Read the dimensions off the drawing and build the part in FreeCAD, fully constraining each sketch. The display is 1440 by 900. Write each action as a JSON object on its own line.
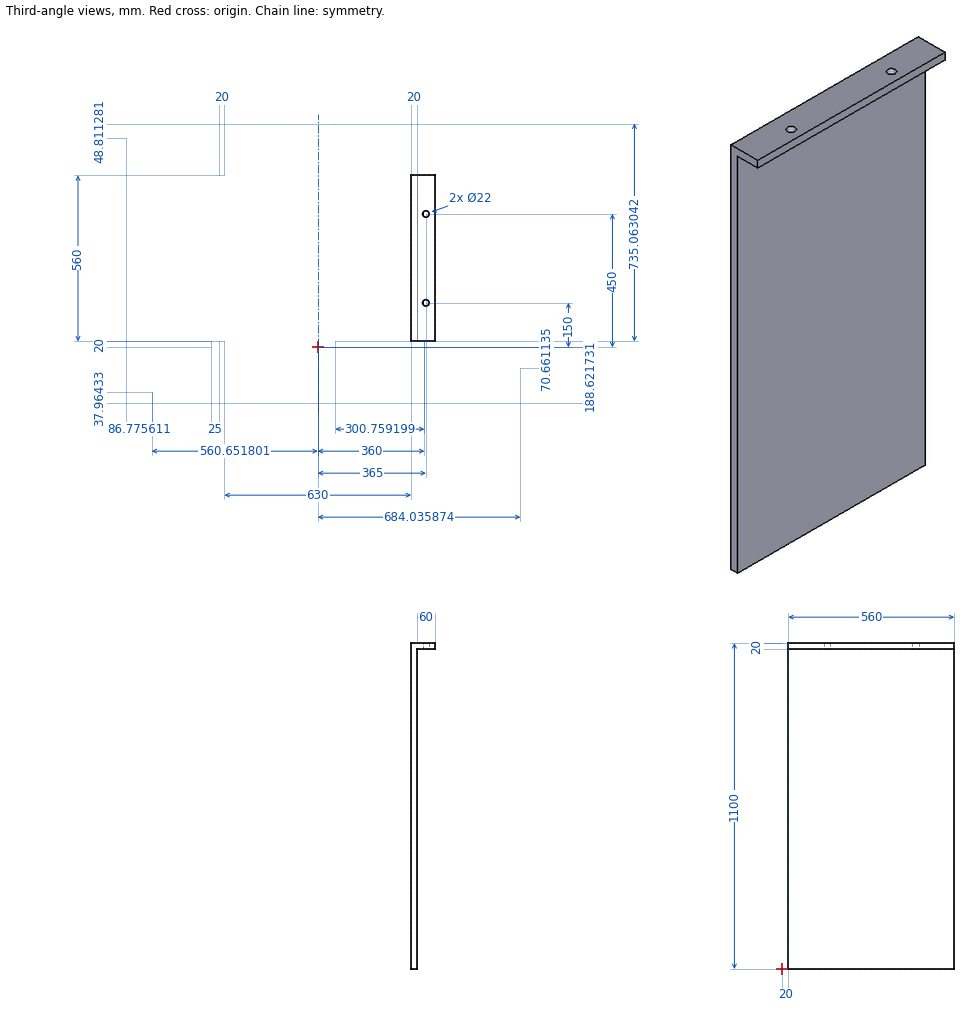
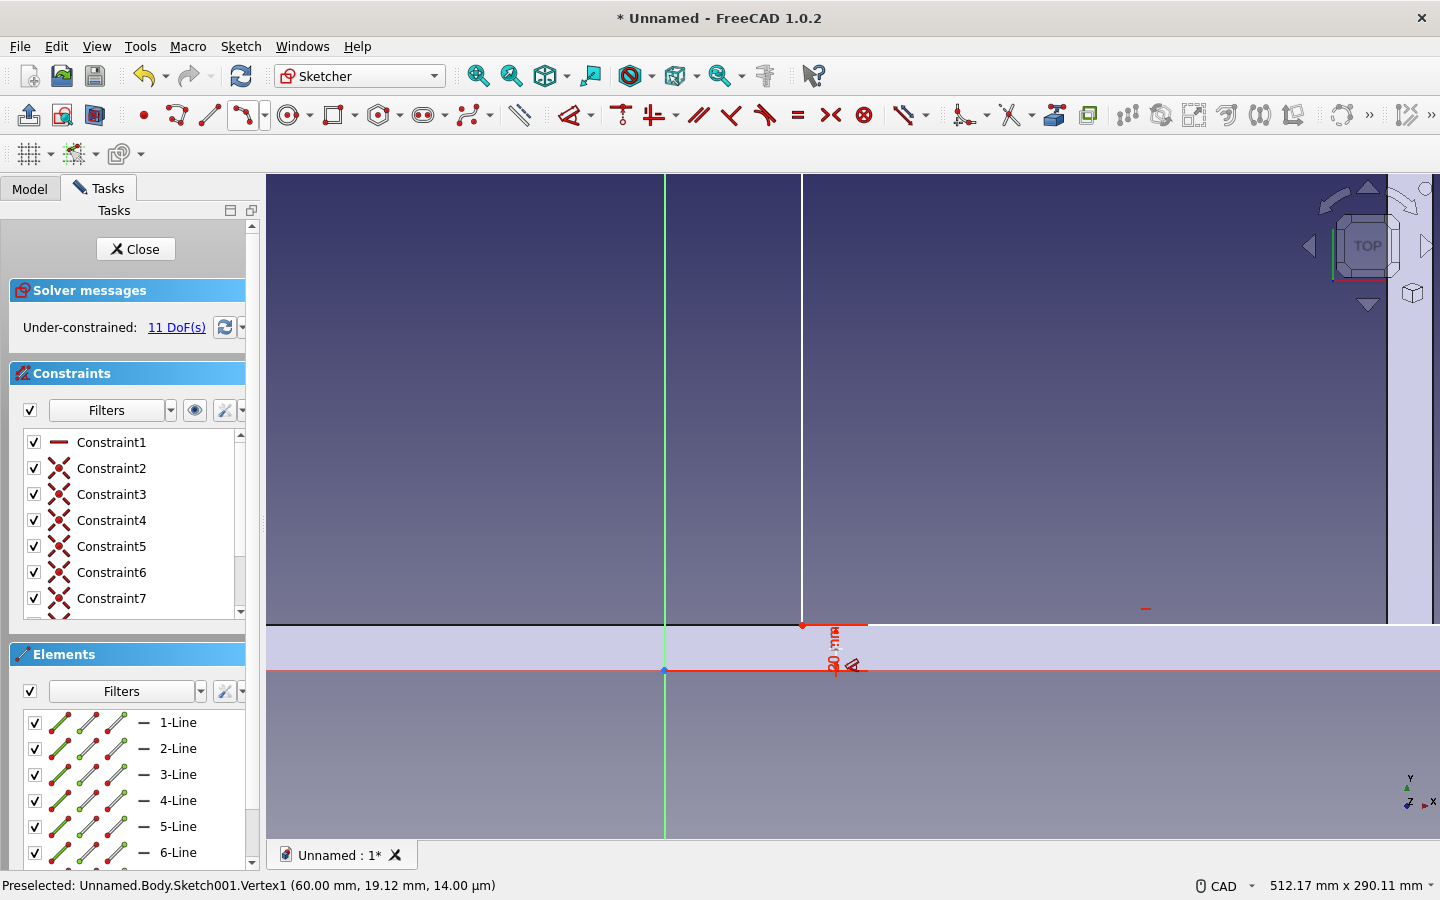
{"action": "scroll", "coordinate": [804, 629], "scroll_direction": "down", "scroll_amount": 8}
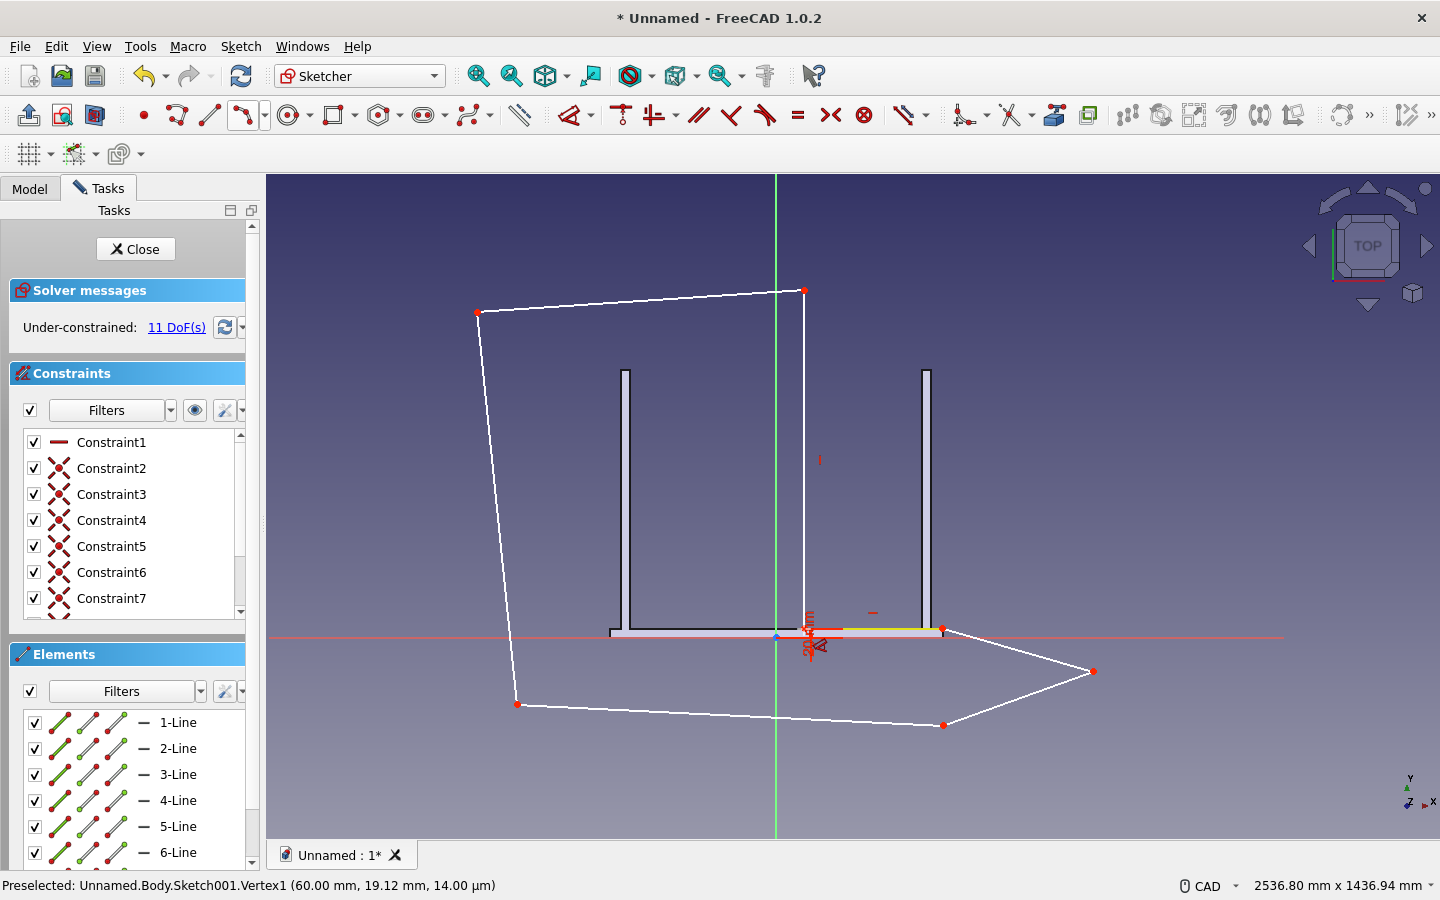
{"action": "left_click", "coordinate": [943, 629]}
{"action": "left_click", "coordinate": [860, 672]}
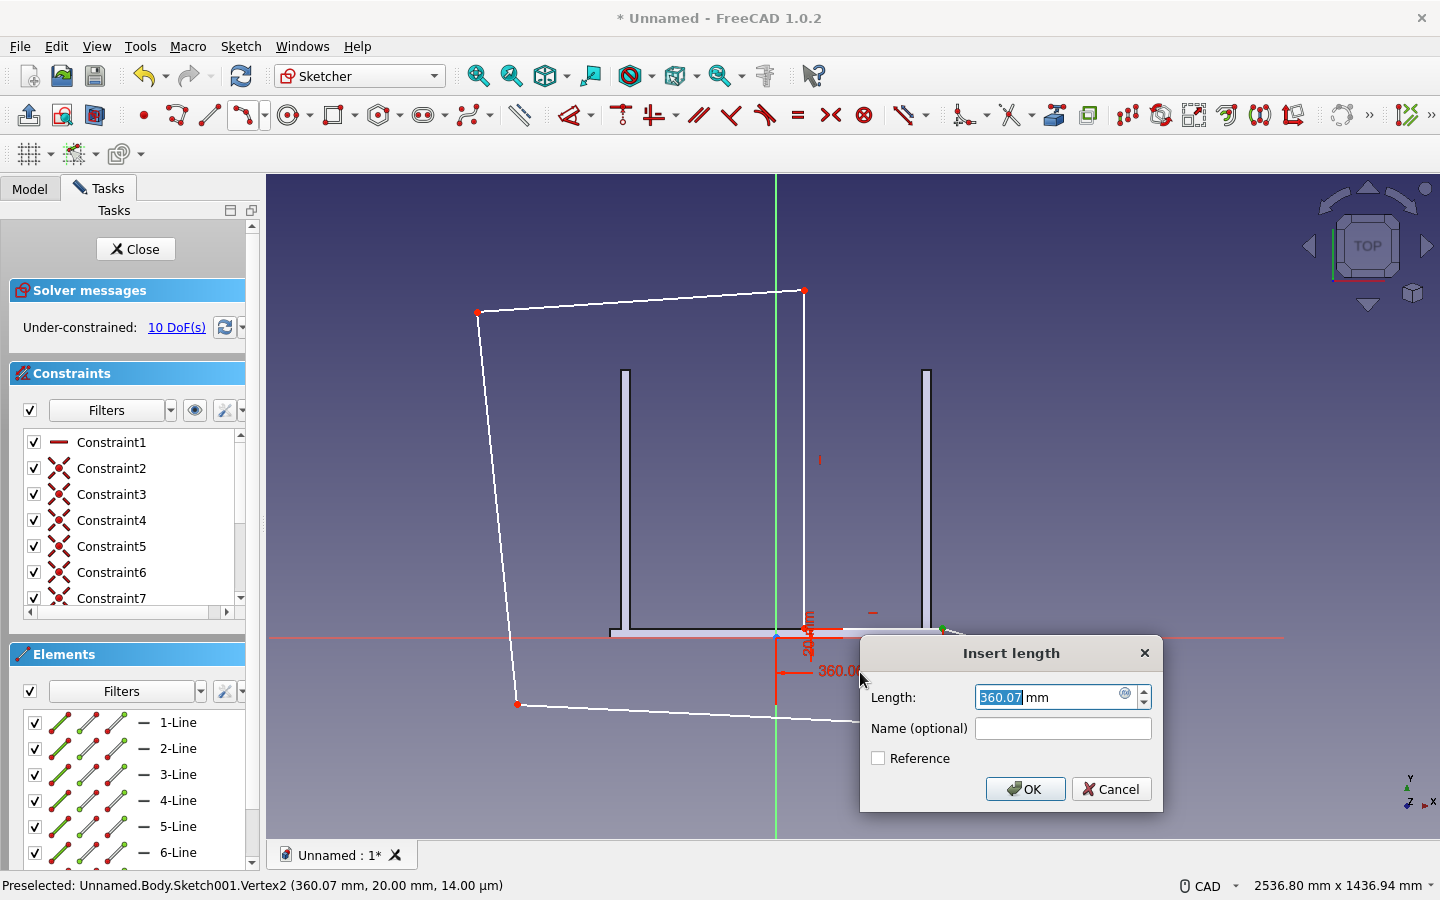
{"action": "type", "text": "360"}
{"action": "key", "text": "Return"}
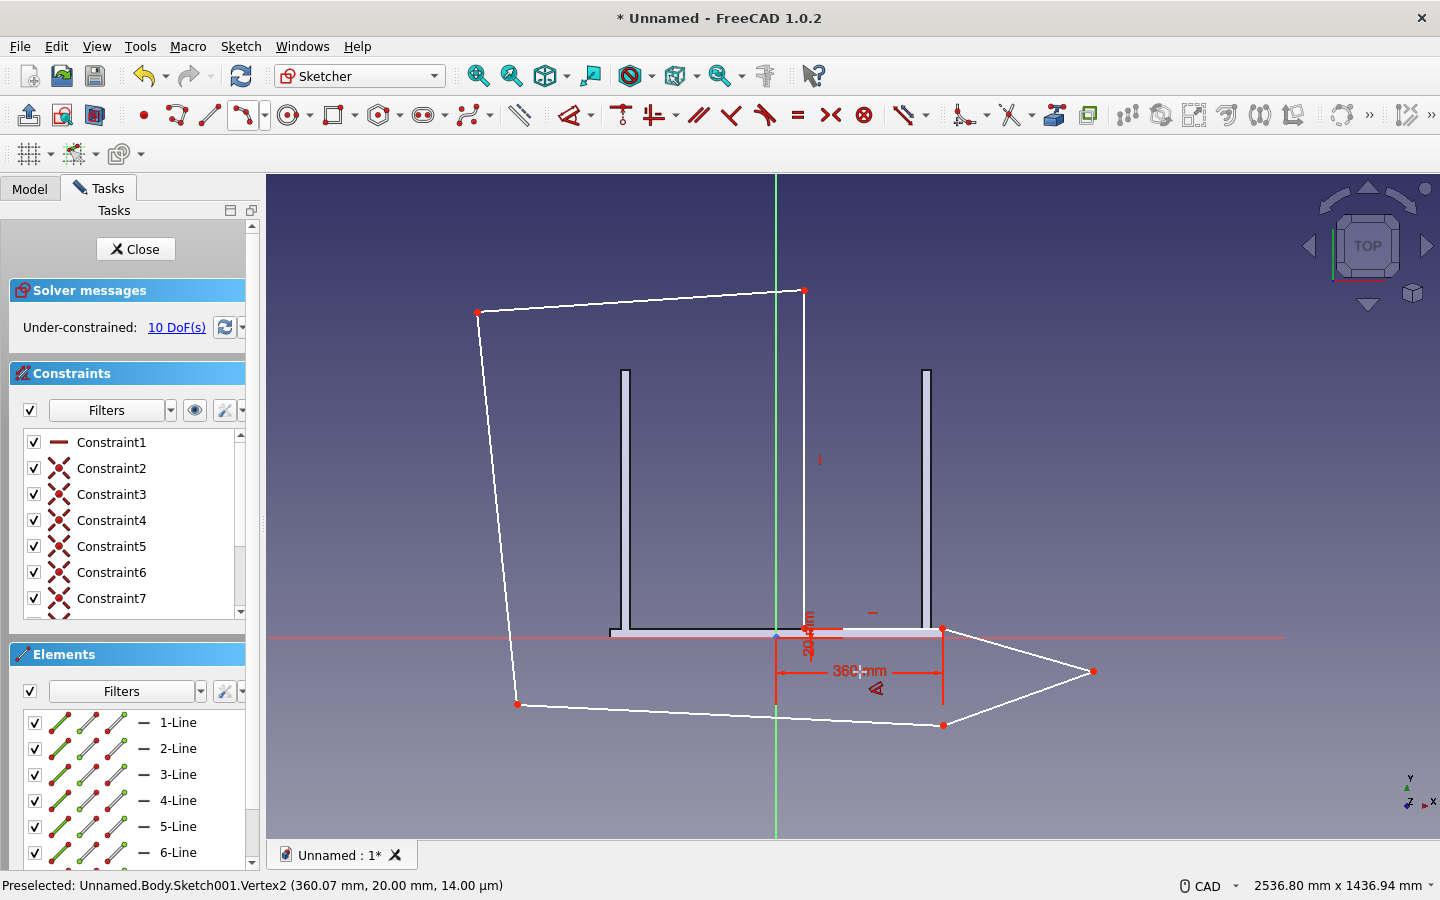
{"action": "left_click", "coordinate": [943, 726]}
{"action": "left_click", "coordinate": [860, 760]}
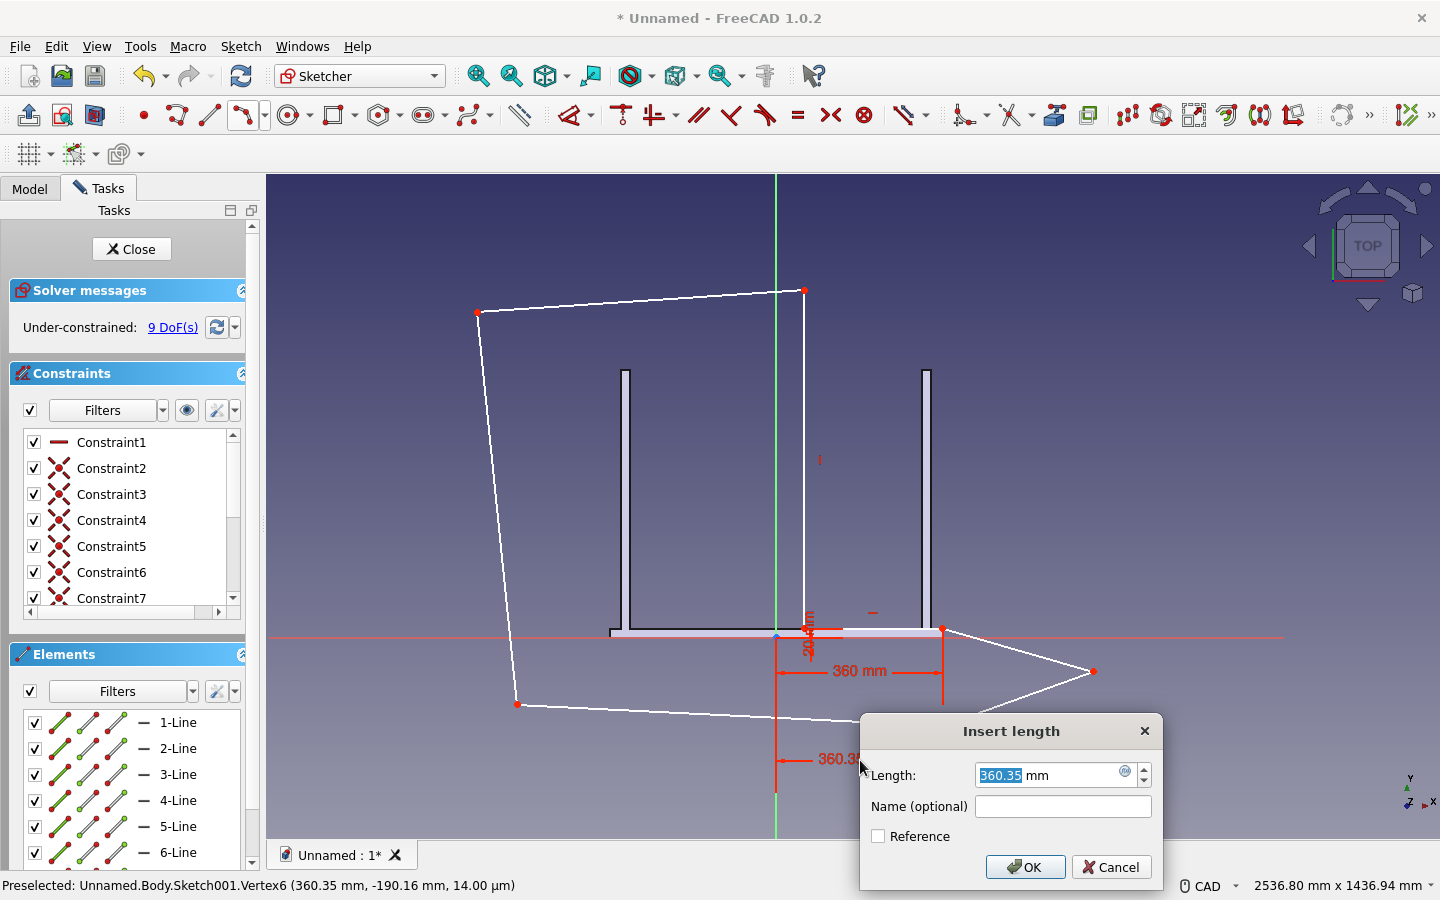
{"action": "type", "text": "360"}
{"action": "key", "text": "Return"}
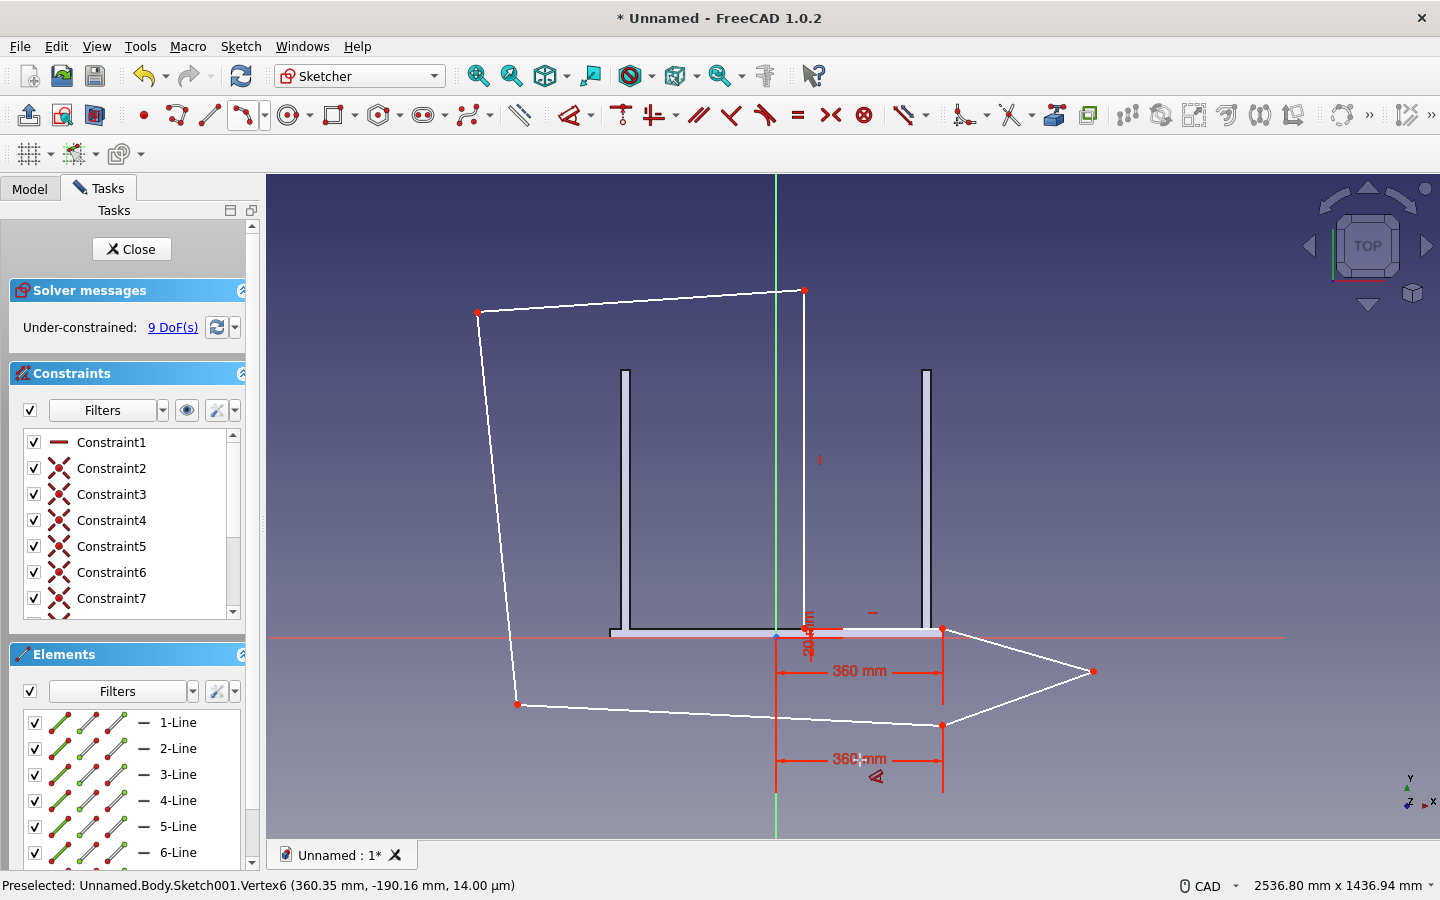
{"action": "scroll", "coordinate": [815, 720], "scroll_direction": "up", "scroll_amount": 5}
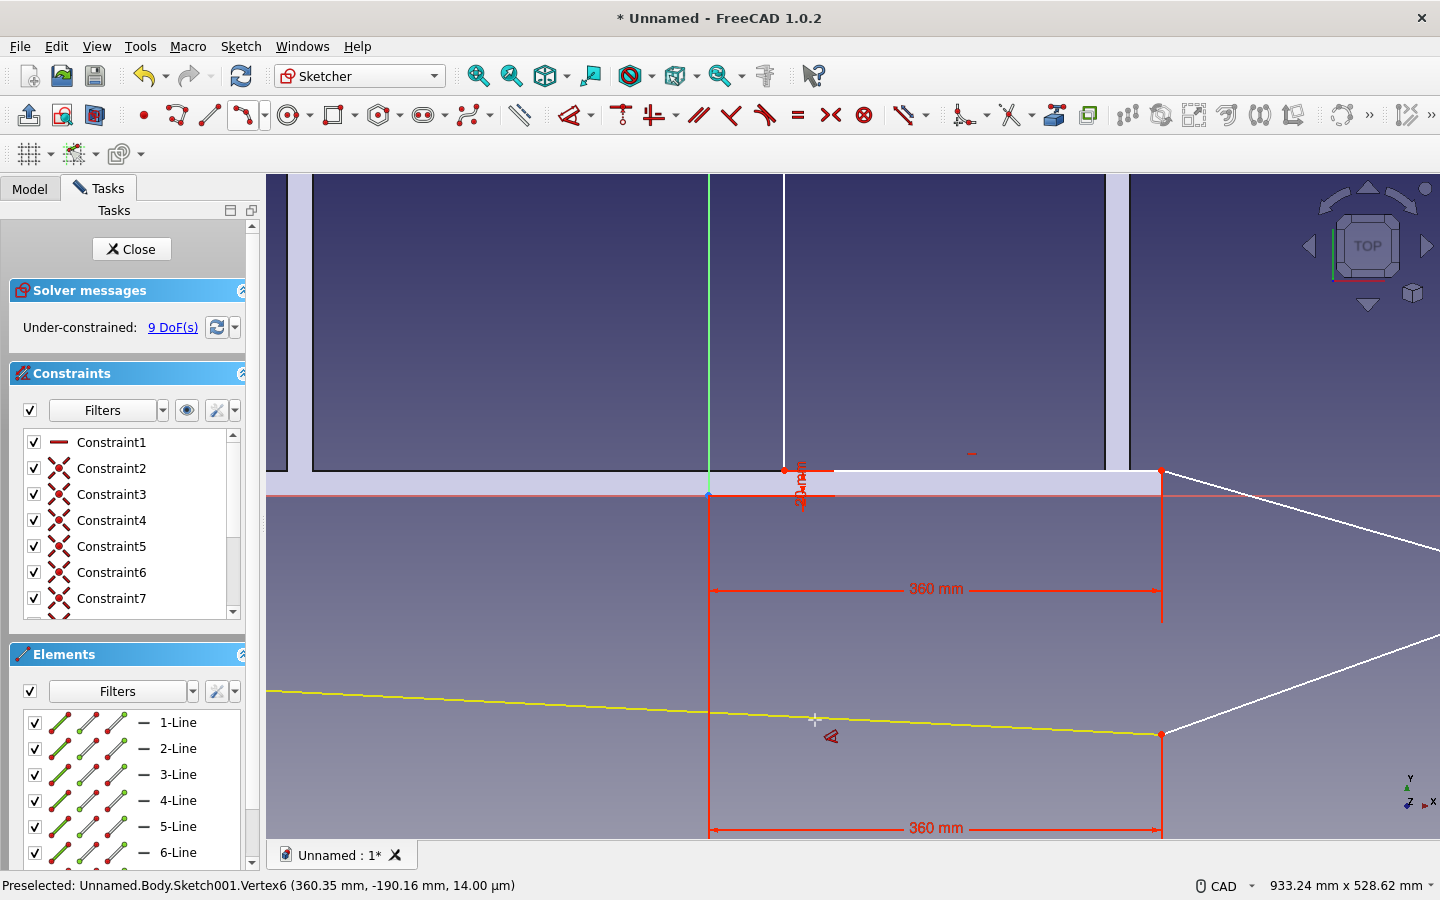
{"action": "left_click", "coordinate": [814, 718]}
{"action": "left_click", "coordinate": [1196, 706]}